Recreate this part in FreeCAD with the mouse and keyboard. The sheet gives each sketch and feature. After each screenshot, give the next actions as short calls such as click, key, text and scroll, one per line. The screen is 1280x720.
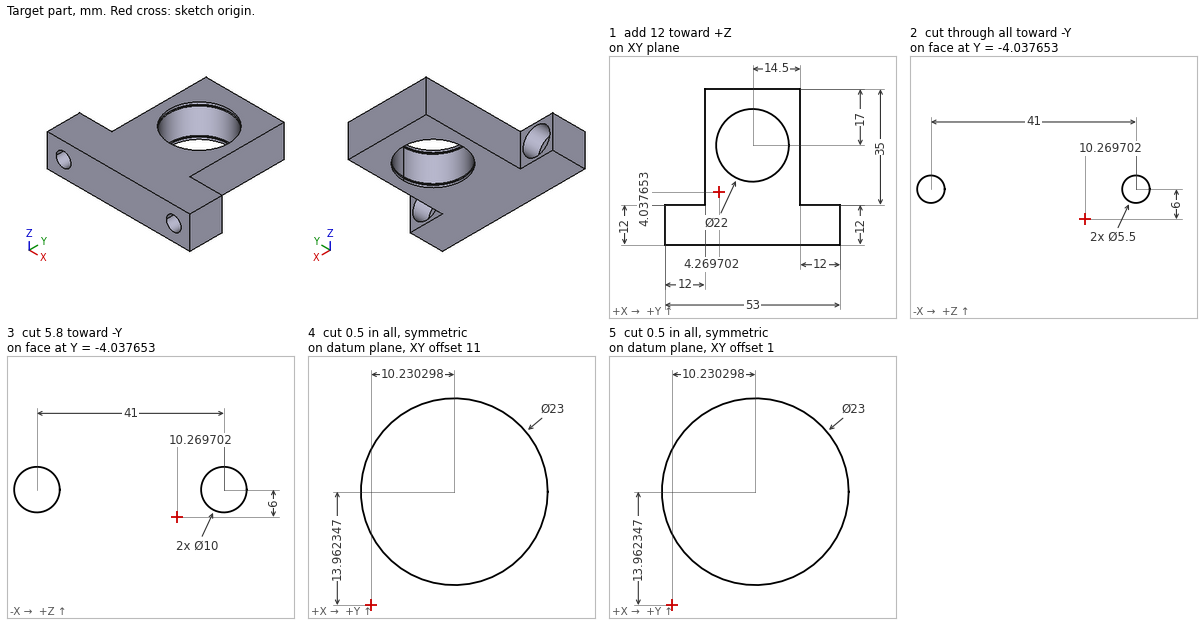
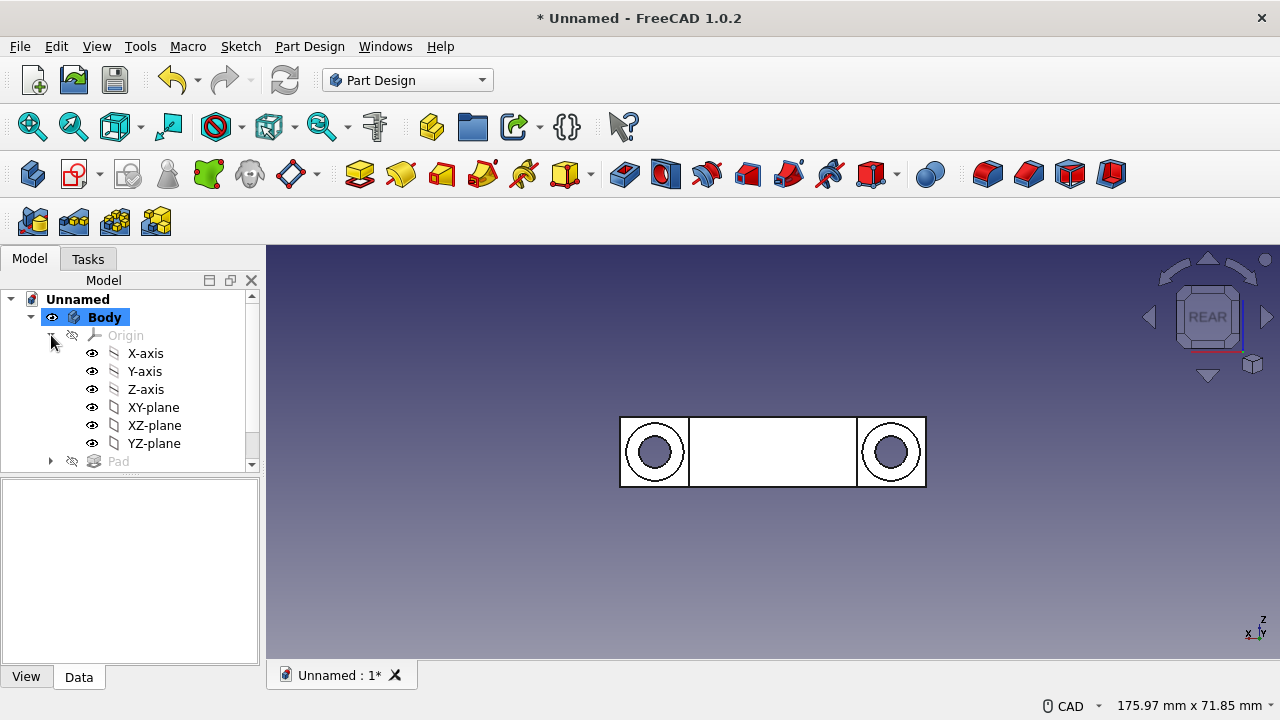
click(137, 407)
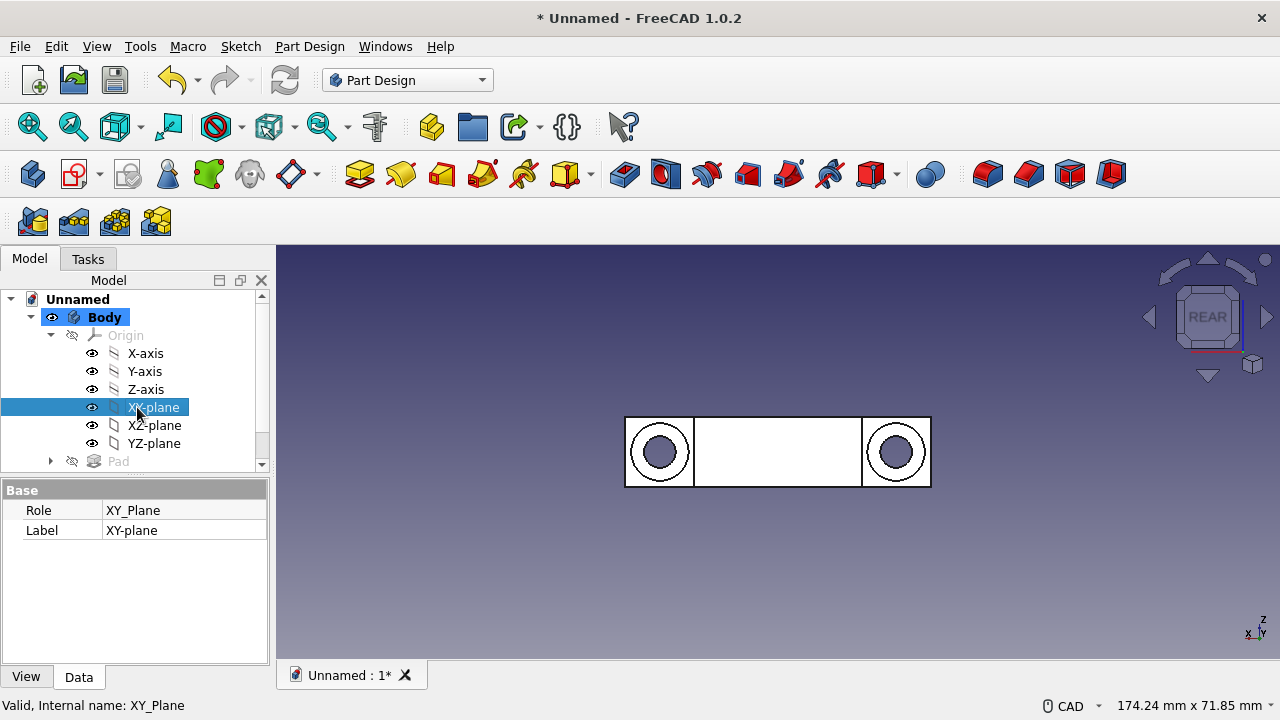
click(290, 174)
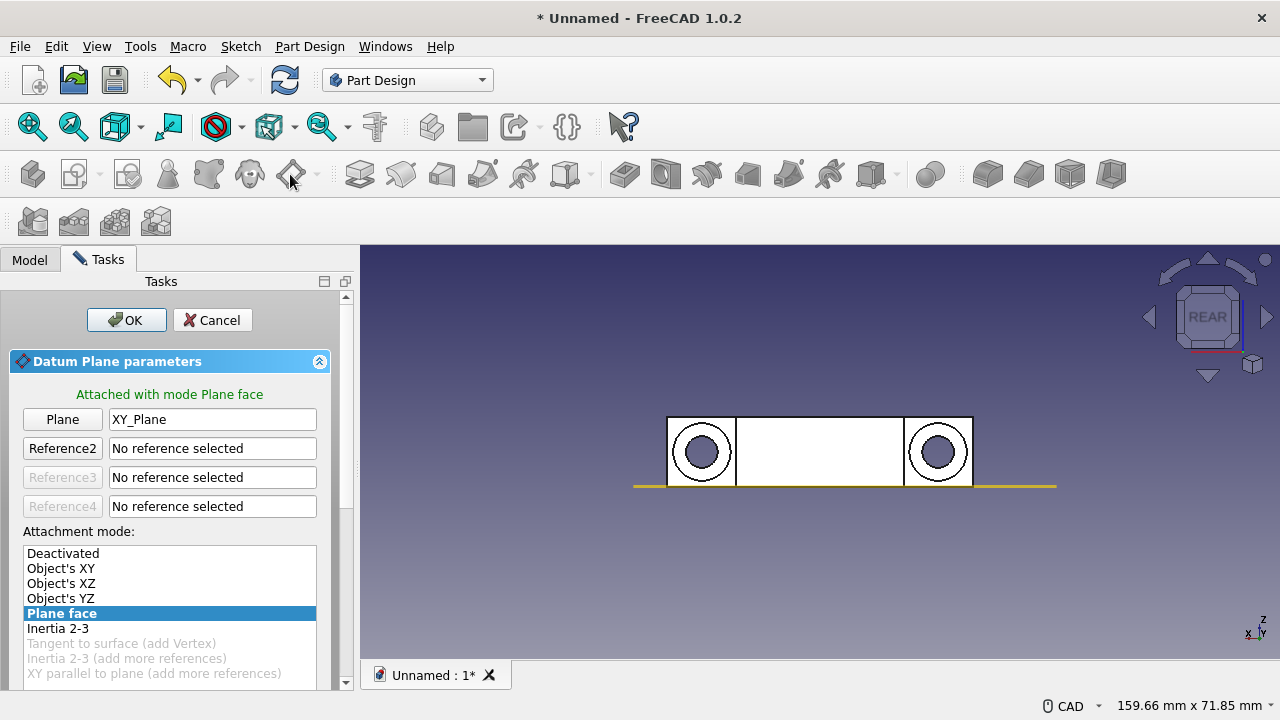
scroll(346, 490, down, 4)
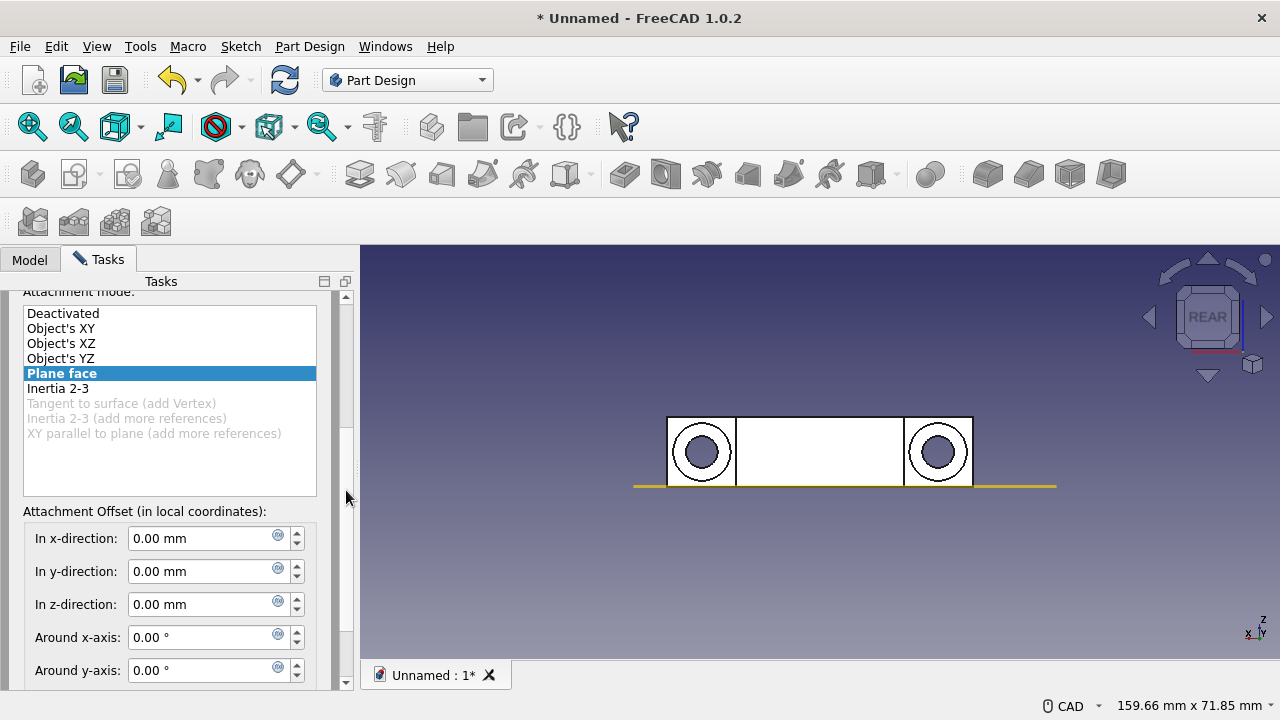
triple_click(210, 604)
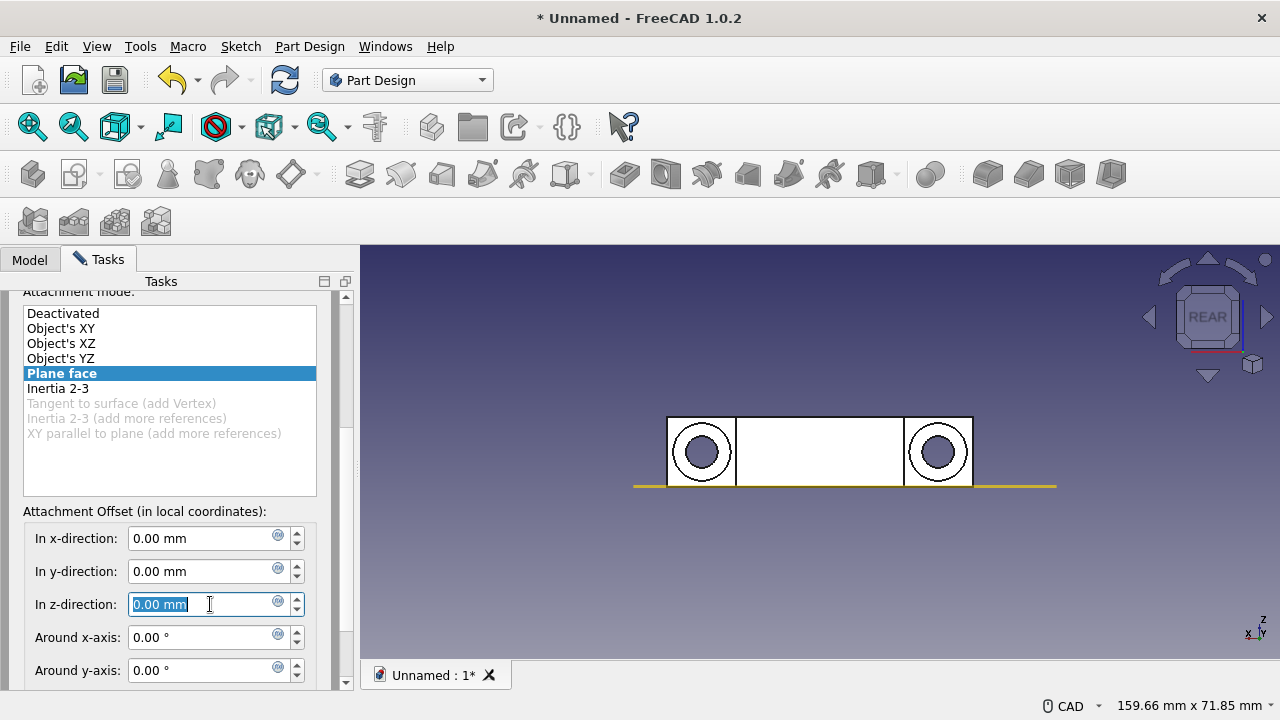
text(11)
key(Tab)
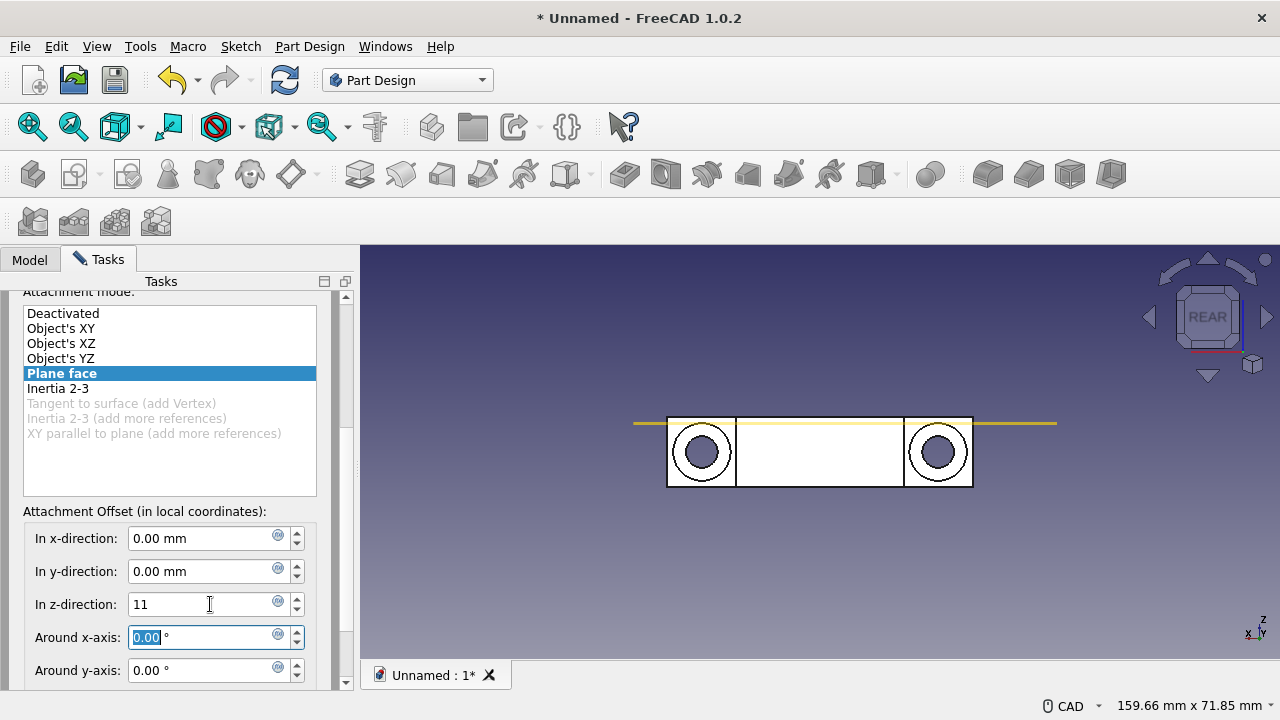
scroll(346, 490, up, 5)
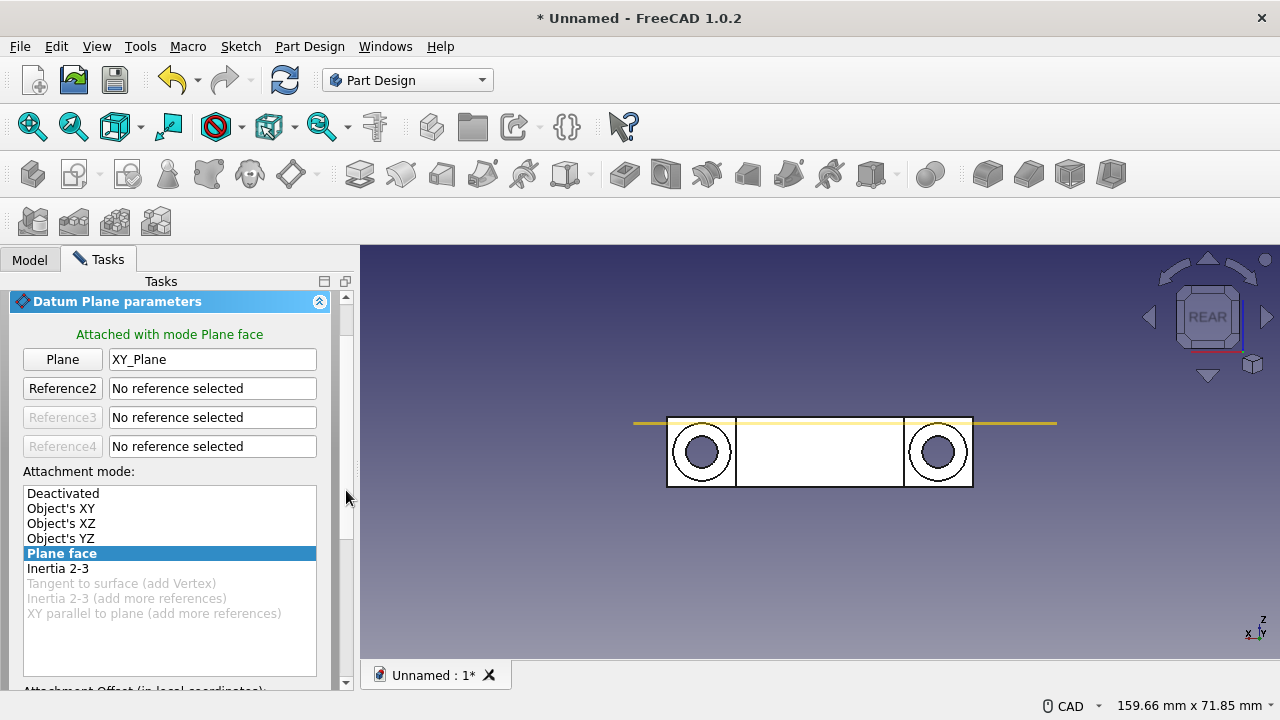
click(127, 320)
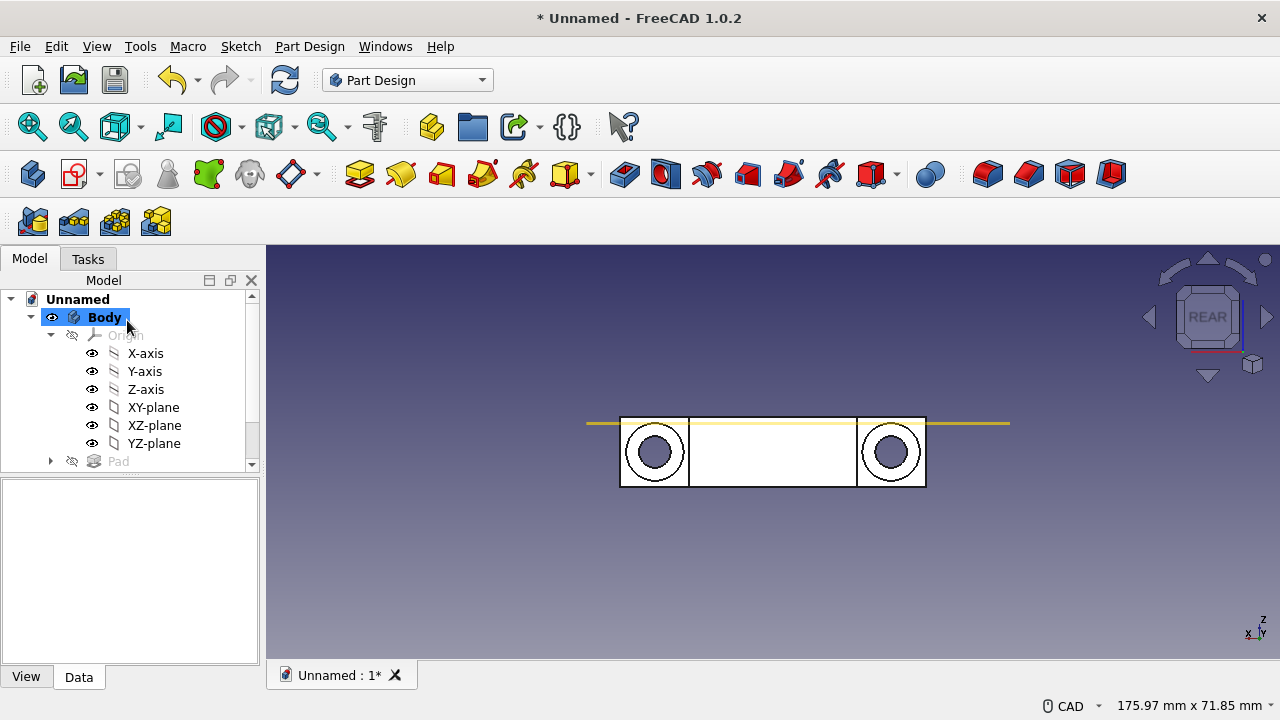
scroll(101, 385, down, 3)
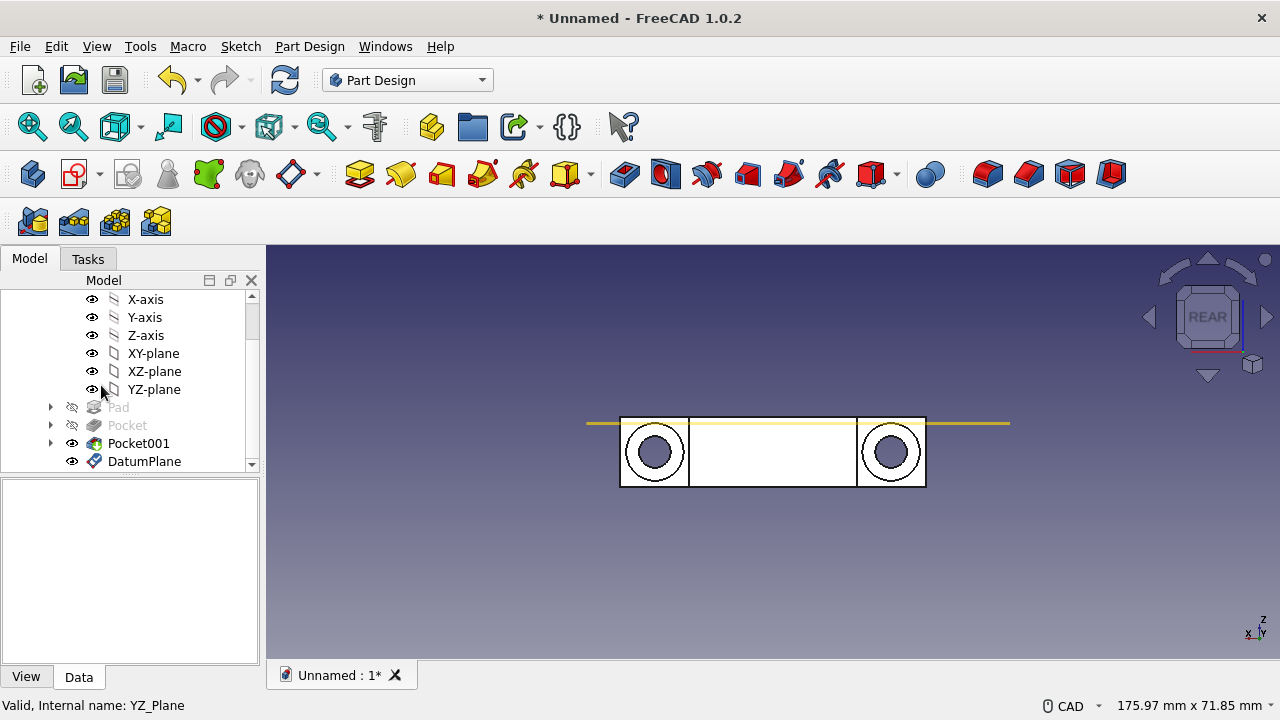
click(117, 461)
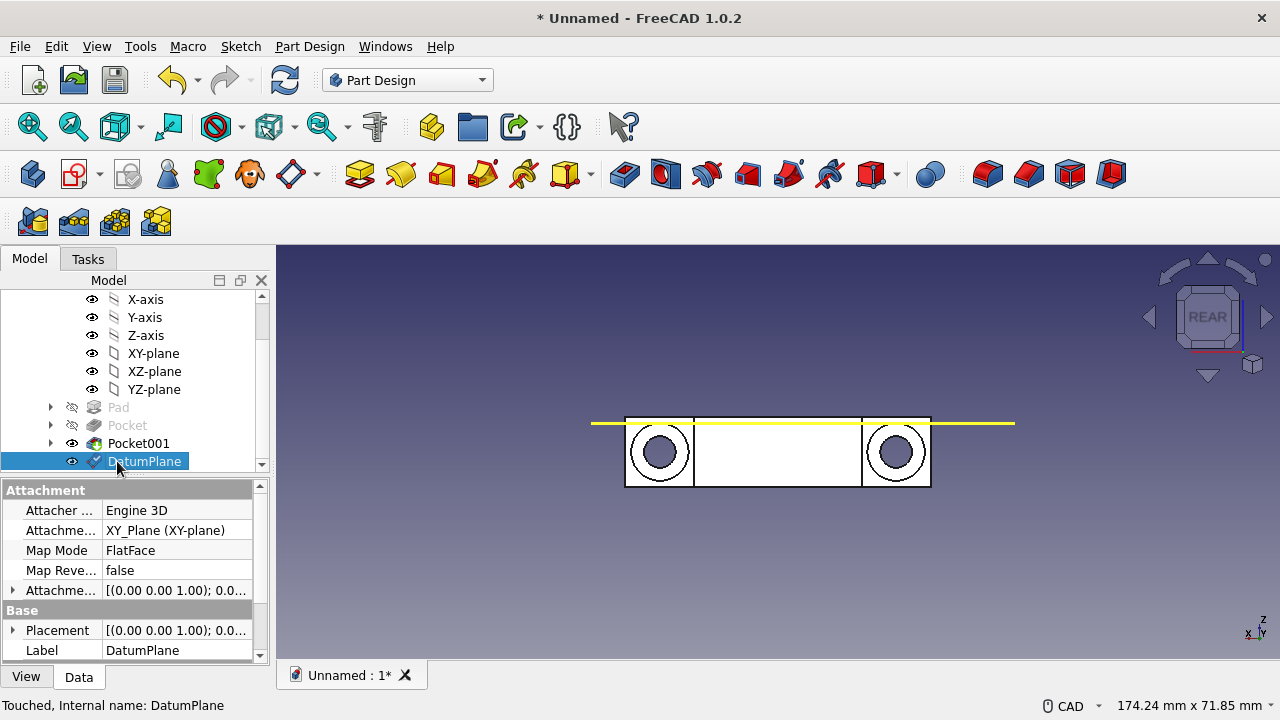
click(74, 174)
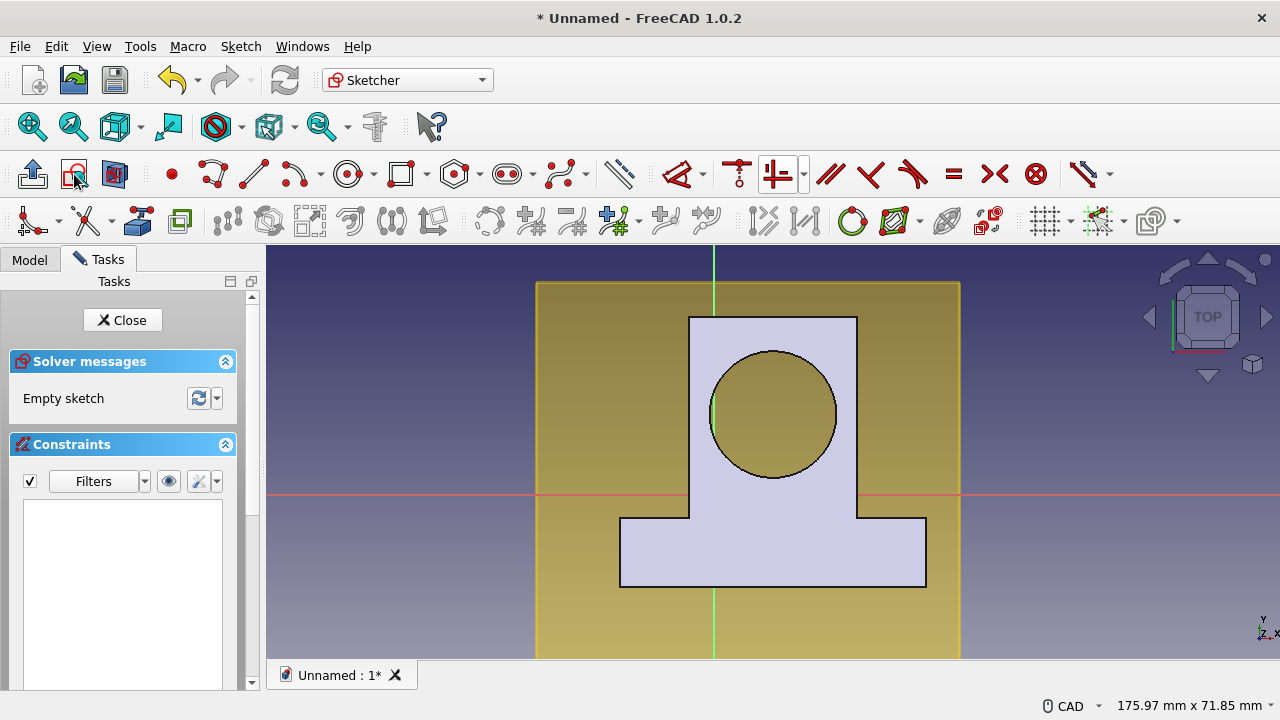
key(q)
key(s)